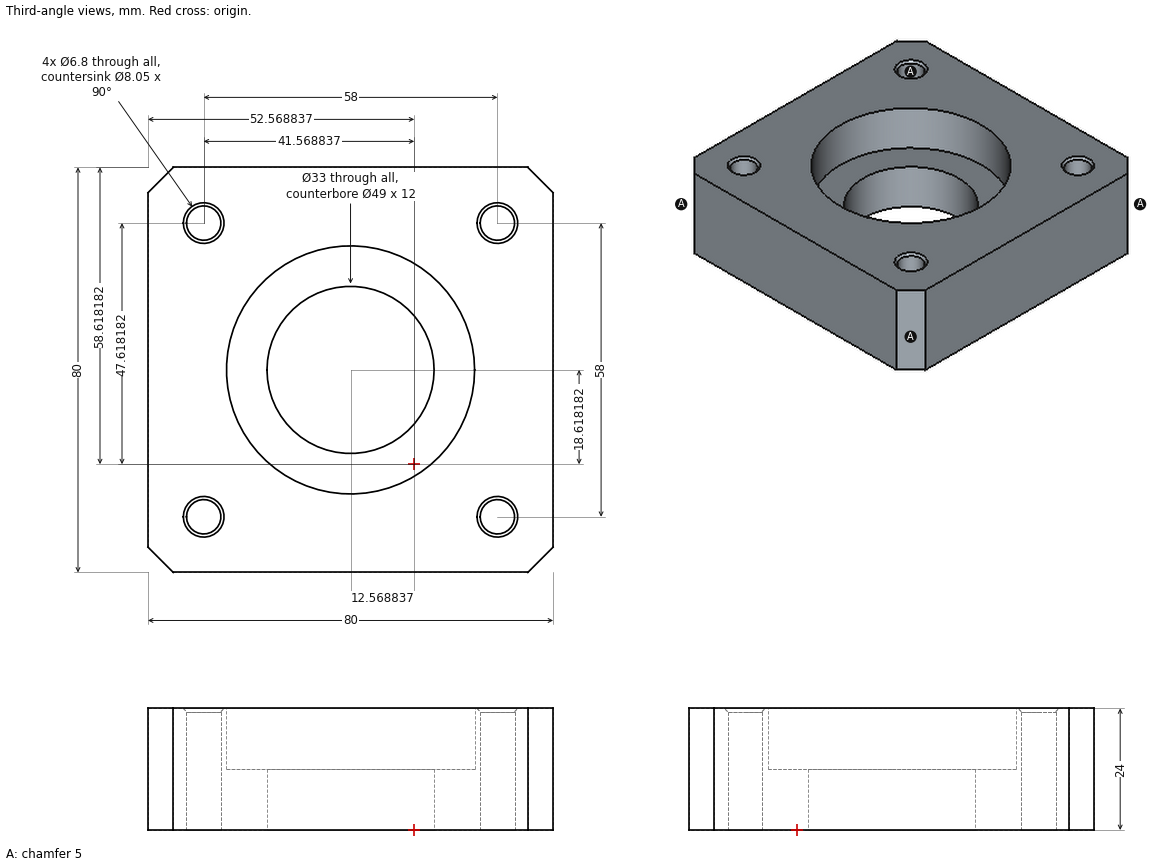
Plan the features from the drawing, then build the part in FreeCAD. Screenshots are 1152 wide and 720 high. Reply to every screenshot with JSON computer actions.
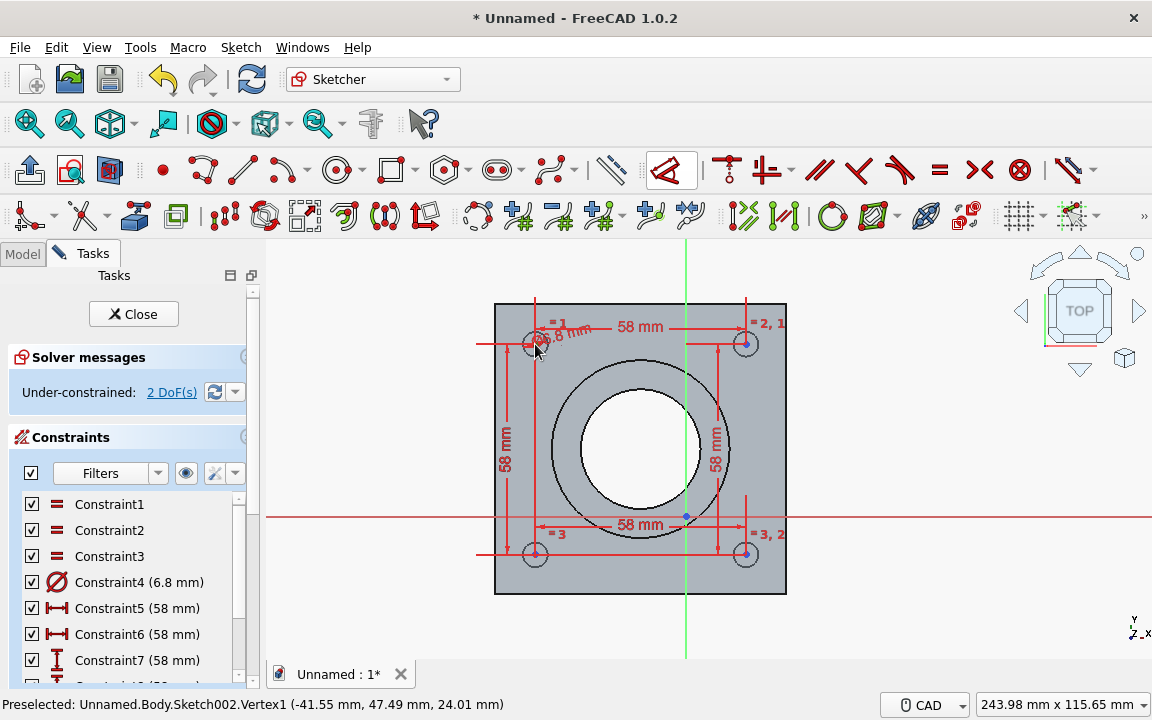
{"action": "key", "text": "l"}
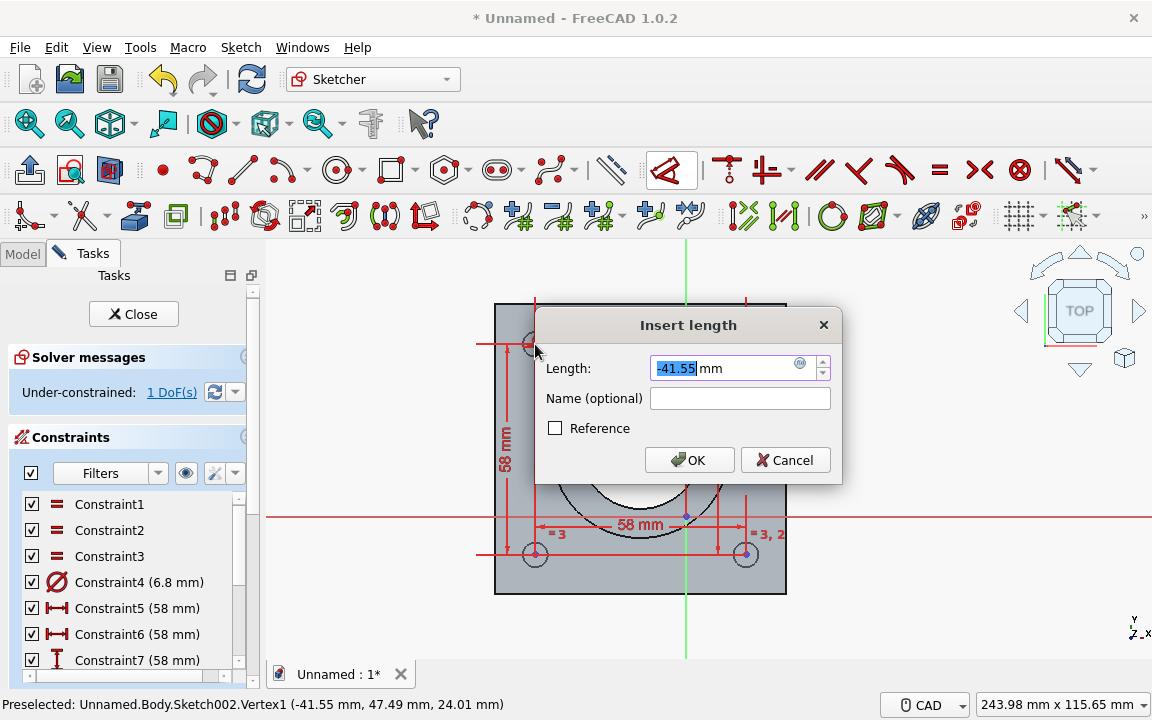
{"action": "type", "text": "-41.568837"}
{"action": "key", "text": "Return"}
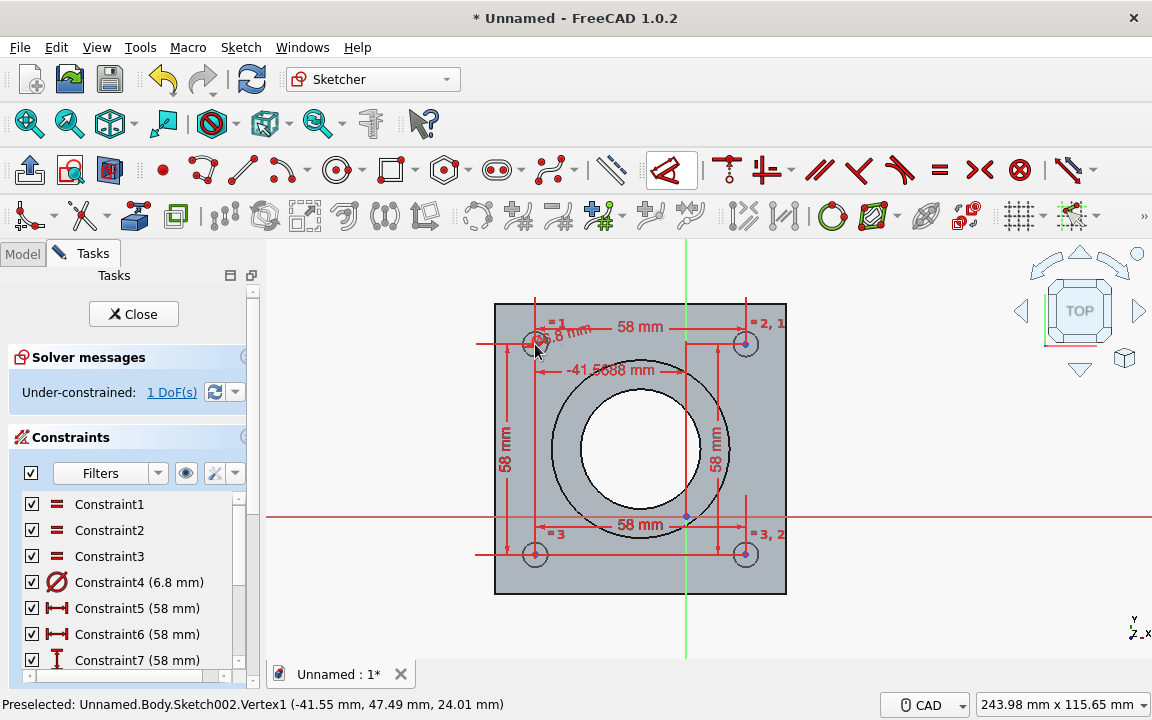
{"action": "left_click", "coordinate": [535, 344]}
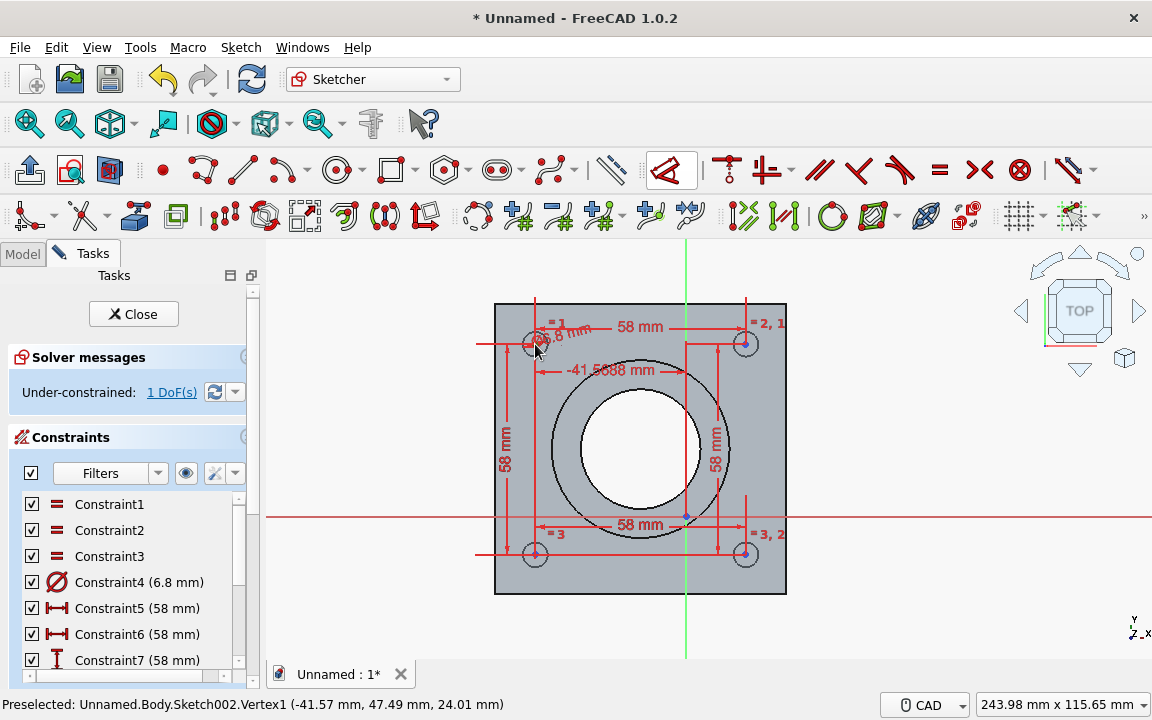
{"action": "key", "text": "i"}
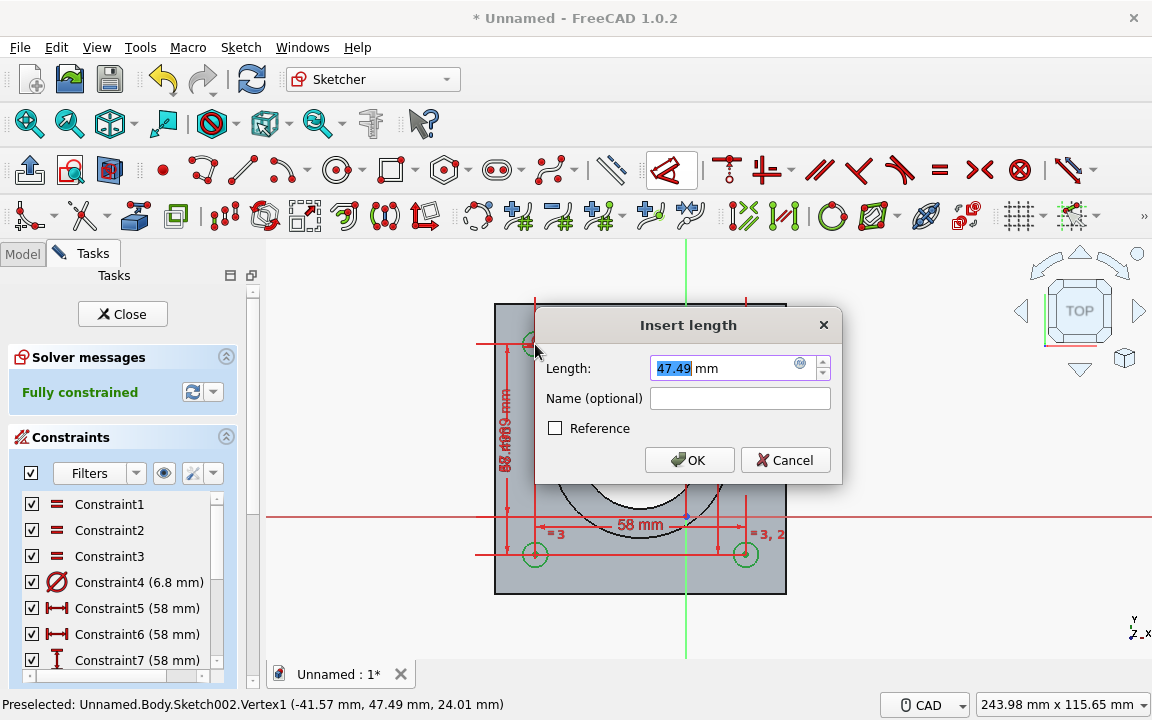
{"action": "type", "text": "47.618182"}
{"action": "key", "text": "Return"}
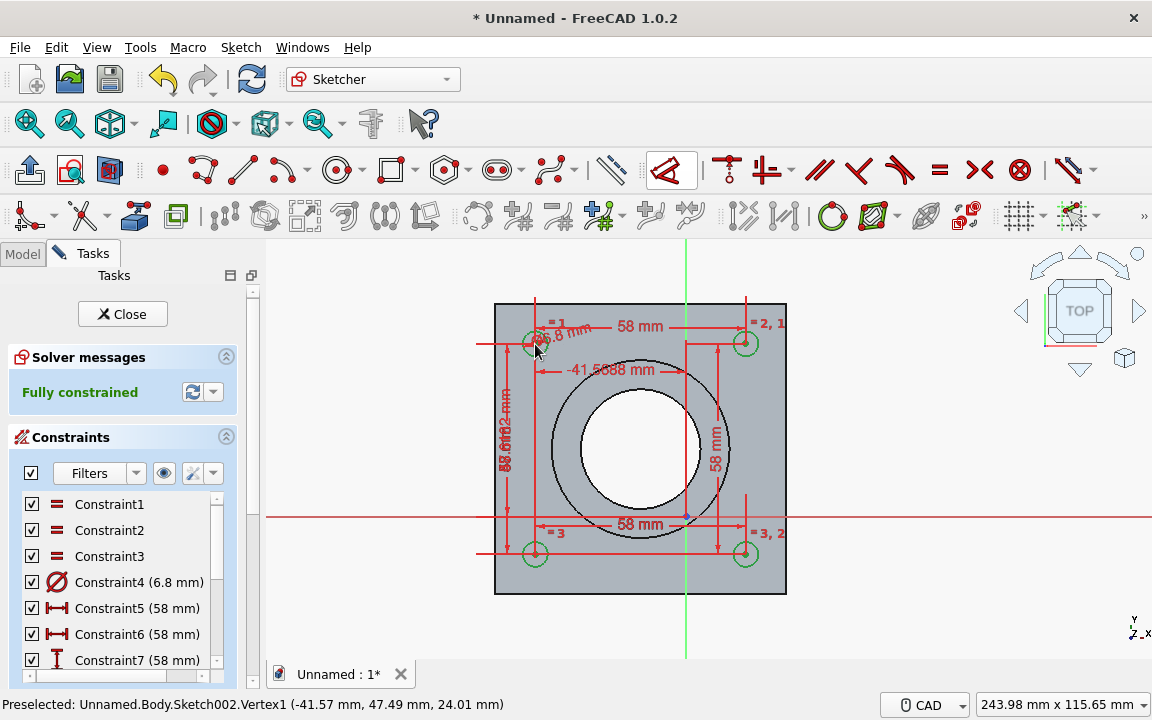
{"action": "left_click", "coordinate": [123, 314]}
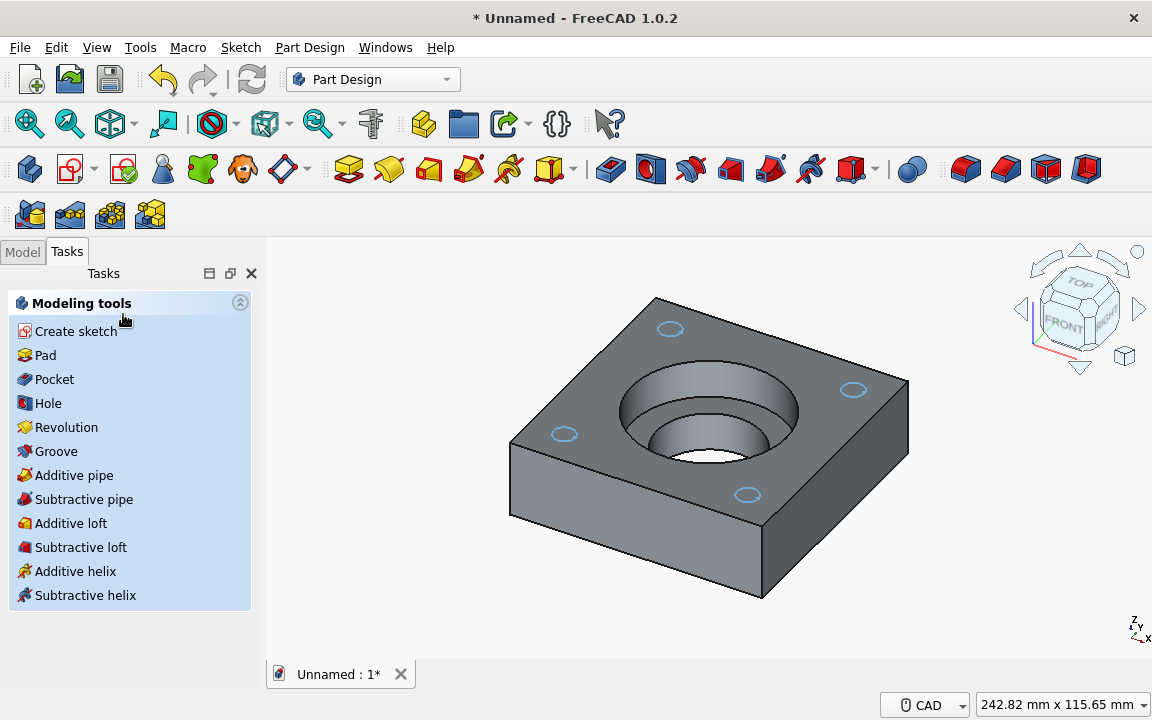
{"action": "left_click", "coordinate": [652, 170]}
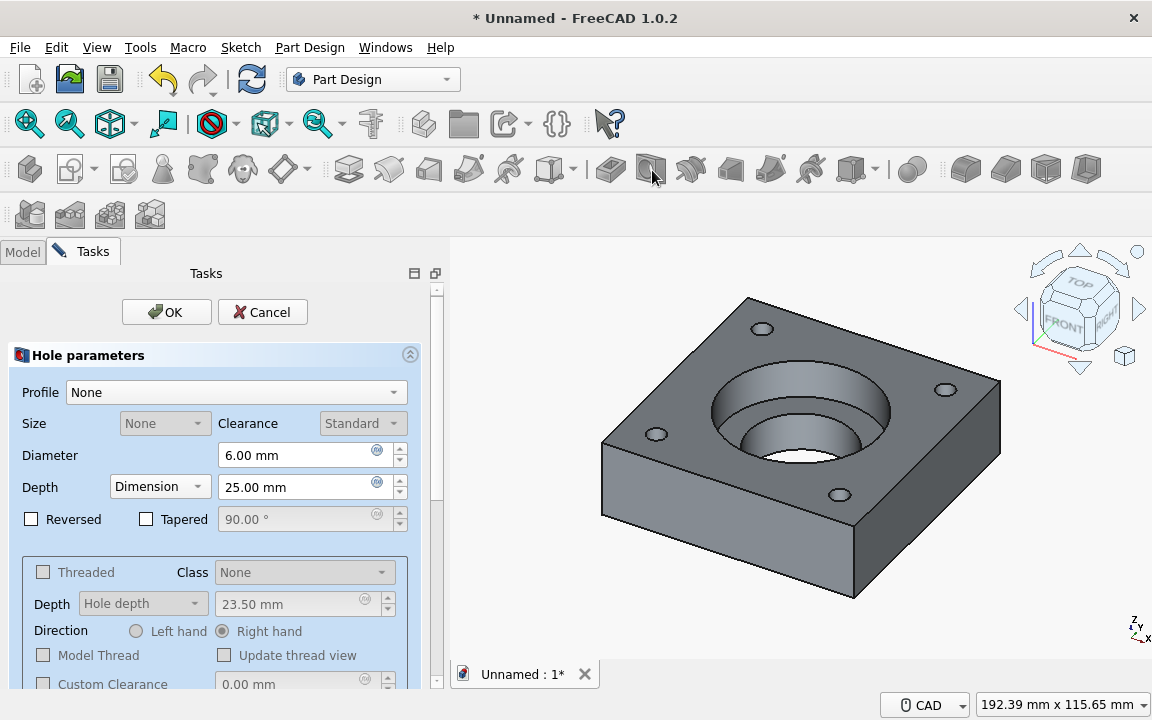
{"action": "triple_click", "coordinate": [305, 455]}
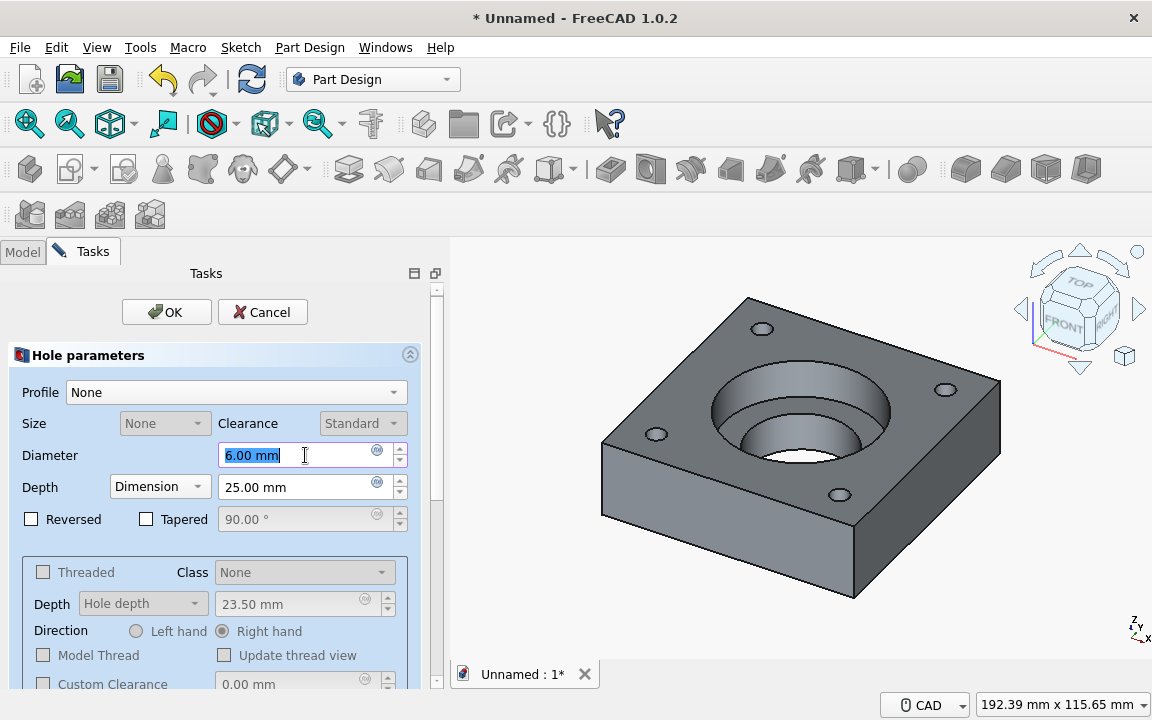
{"action": "type", "text": "6.8"}
{"action": "key", "text": "Tab"}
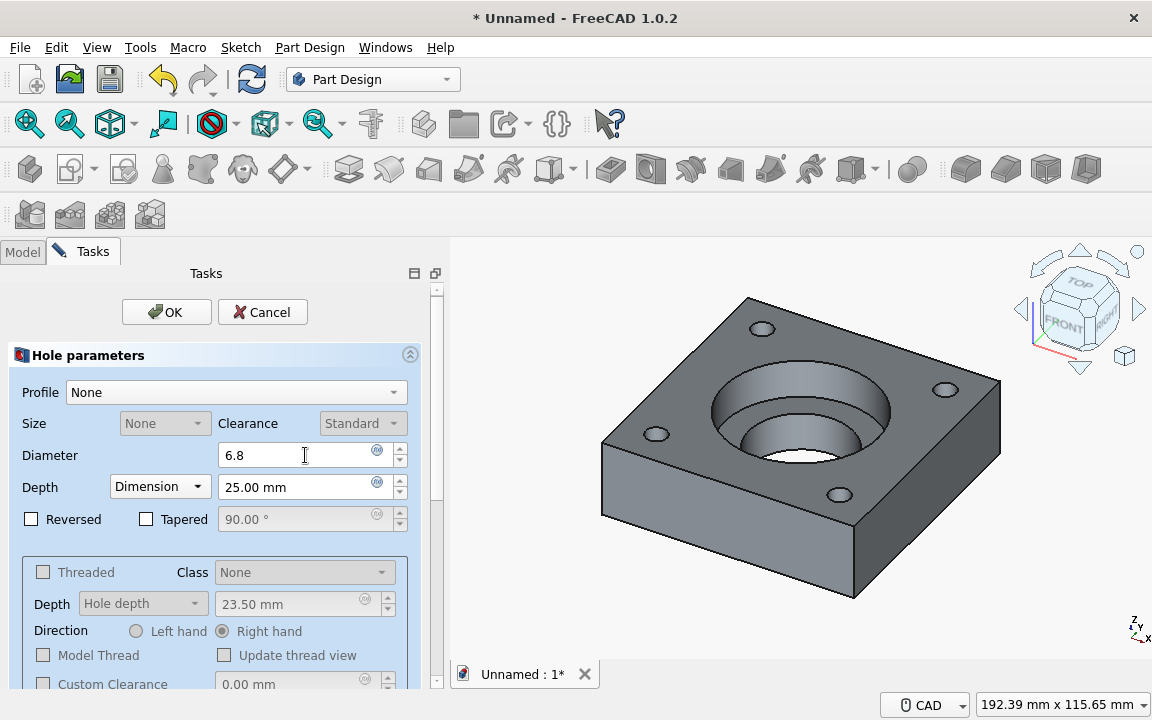
{"action": "left_click", "coordinate": [161, 486]}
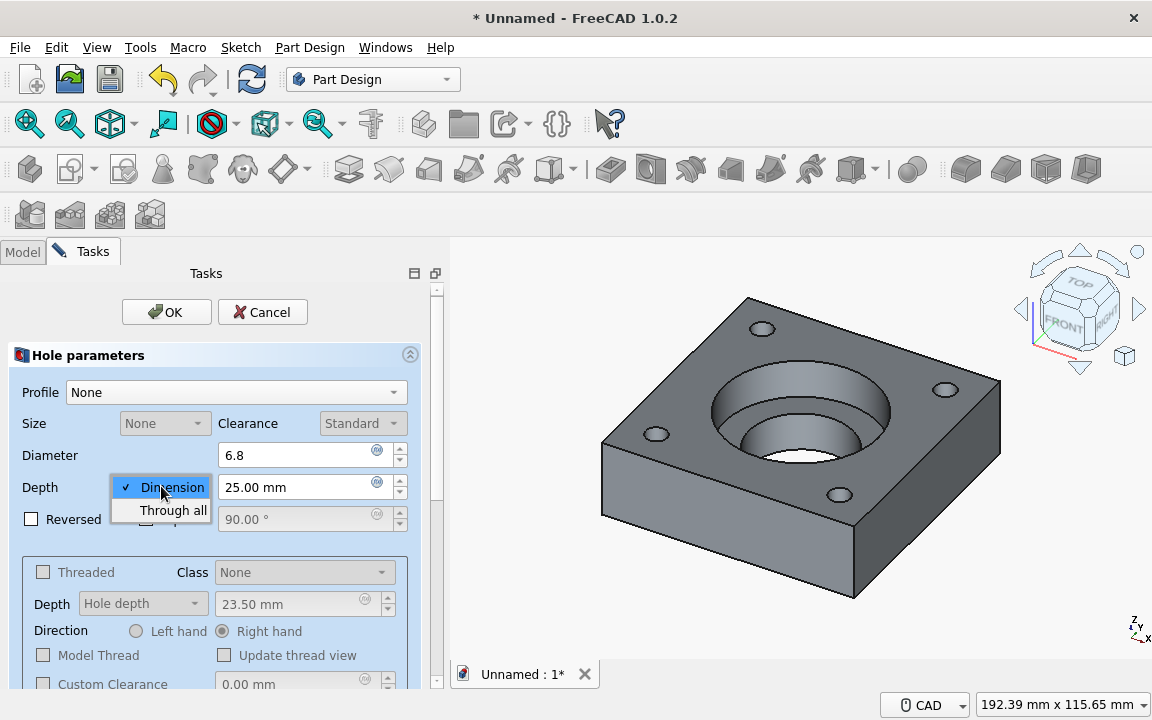
{"action": "left_click", "coordinate": [160, 510]}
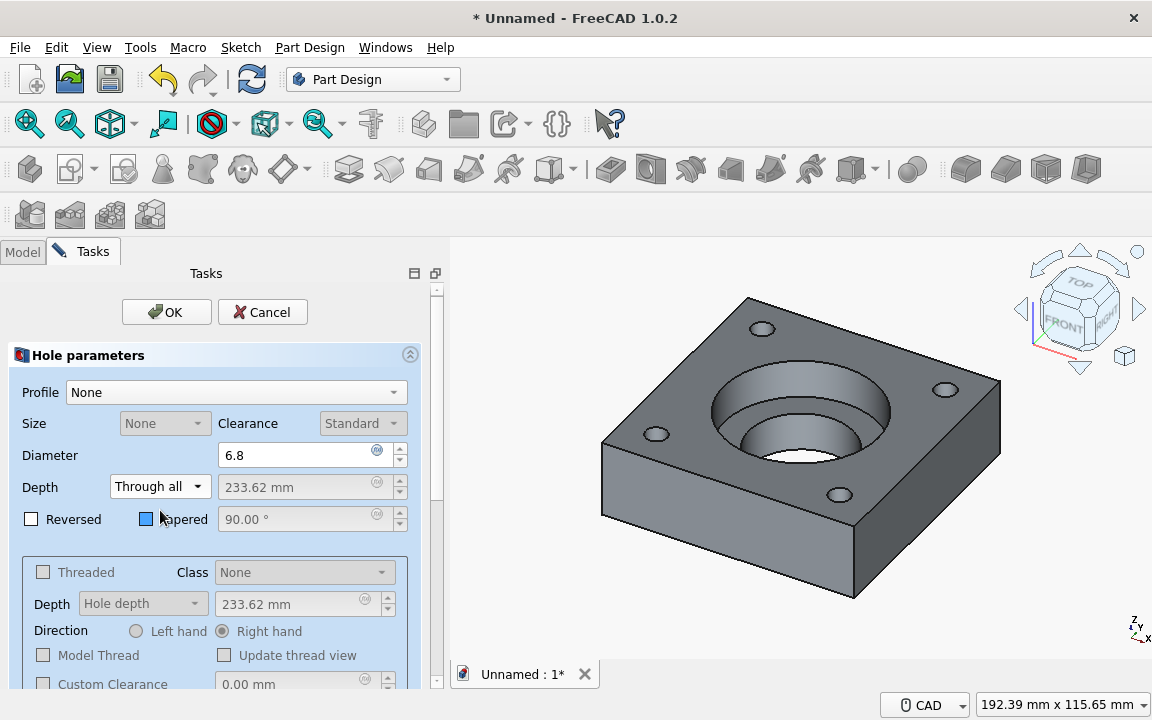
{"action": "scroll", "coordinate": [437, 486], "scroll_direction": "down", "scroll_amount": 3}